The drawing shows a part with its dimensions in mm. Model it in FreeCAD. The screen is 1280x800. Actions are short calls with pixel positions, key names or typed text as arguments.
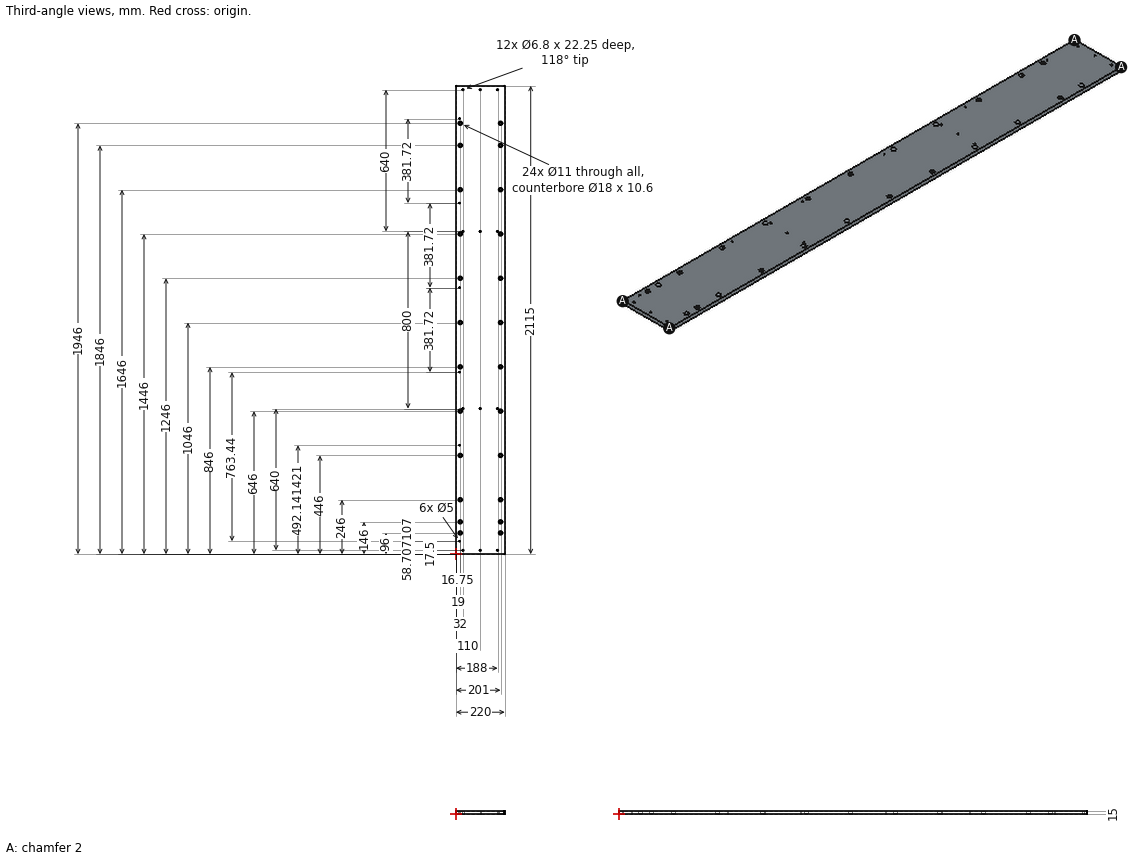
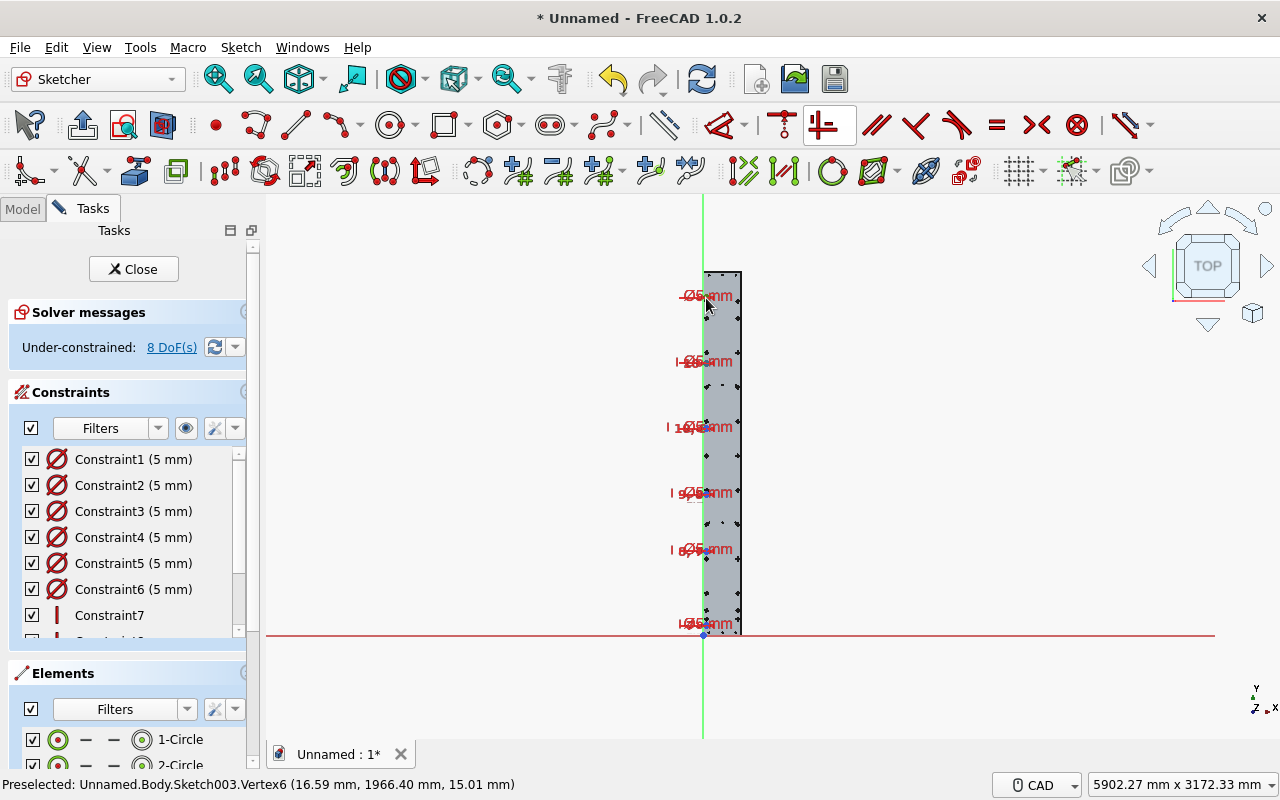
key(v)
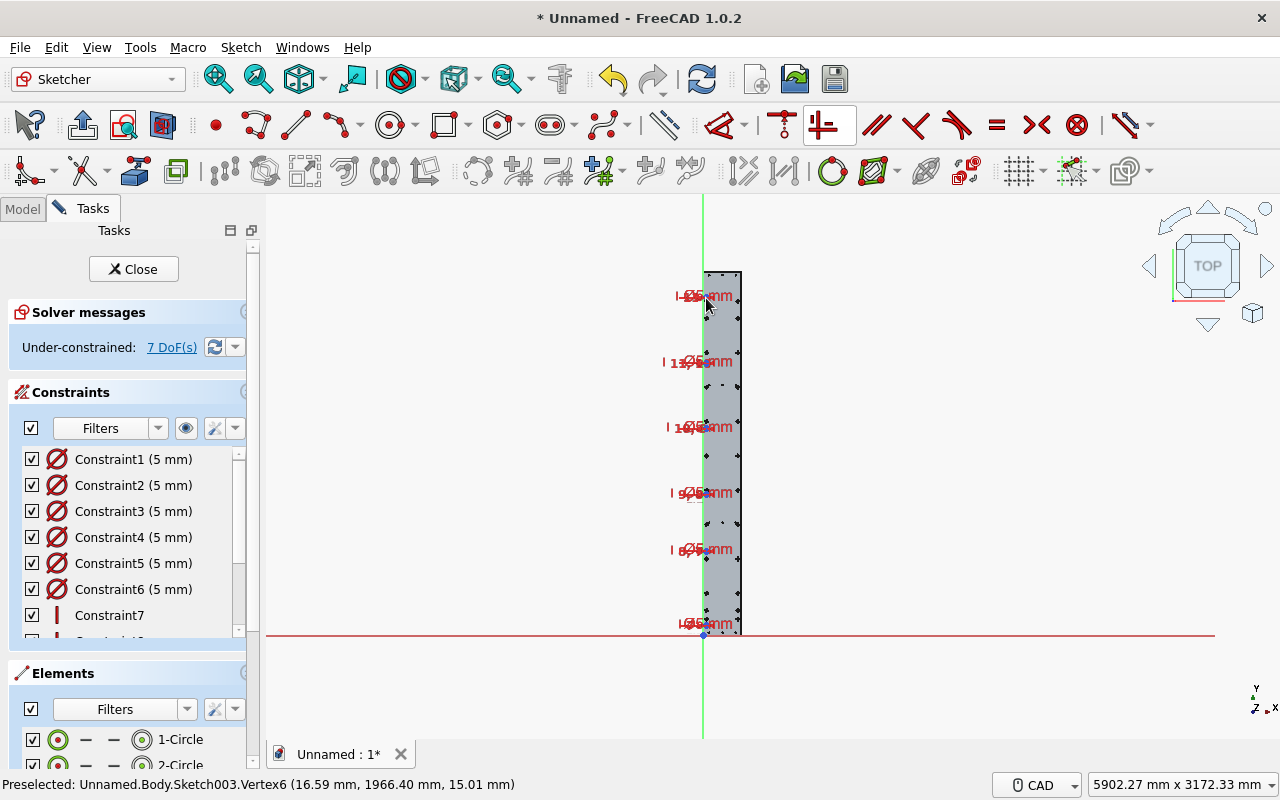
click(720, 126)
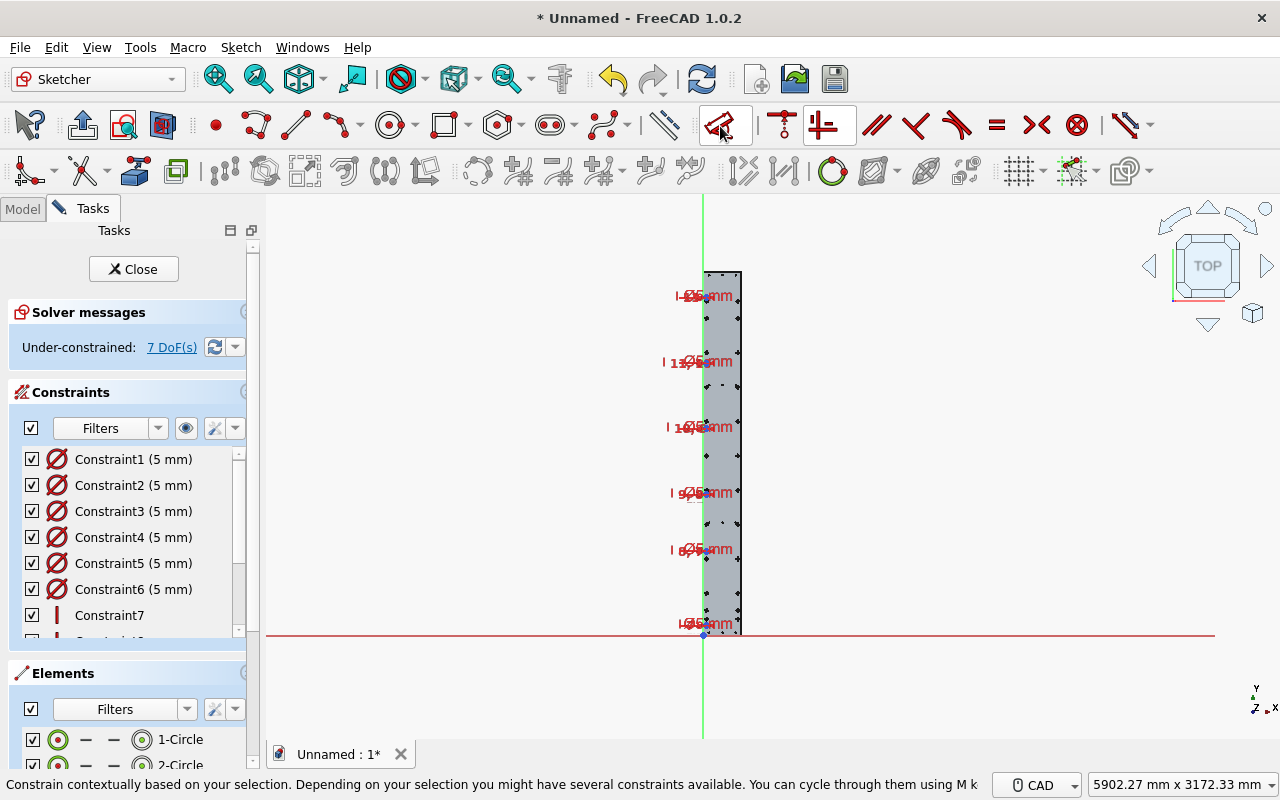
scroll(706, 626, up, 14)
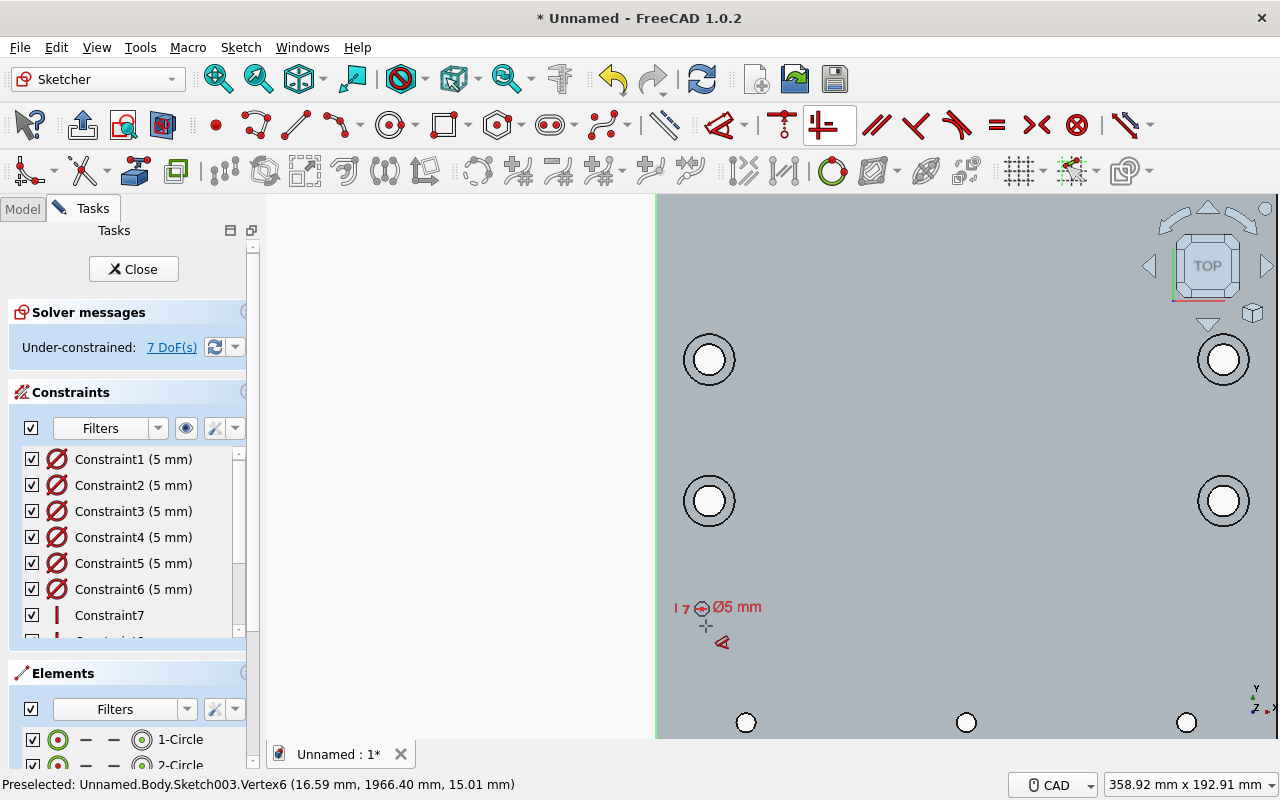
click(702, 609)
click(679, 575)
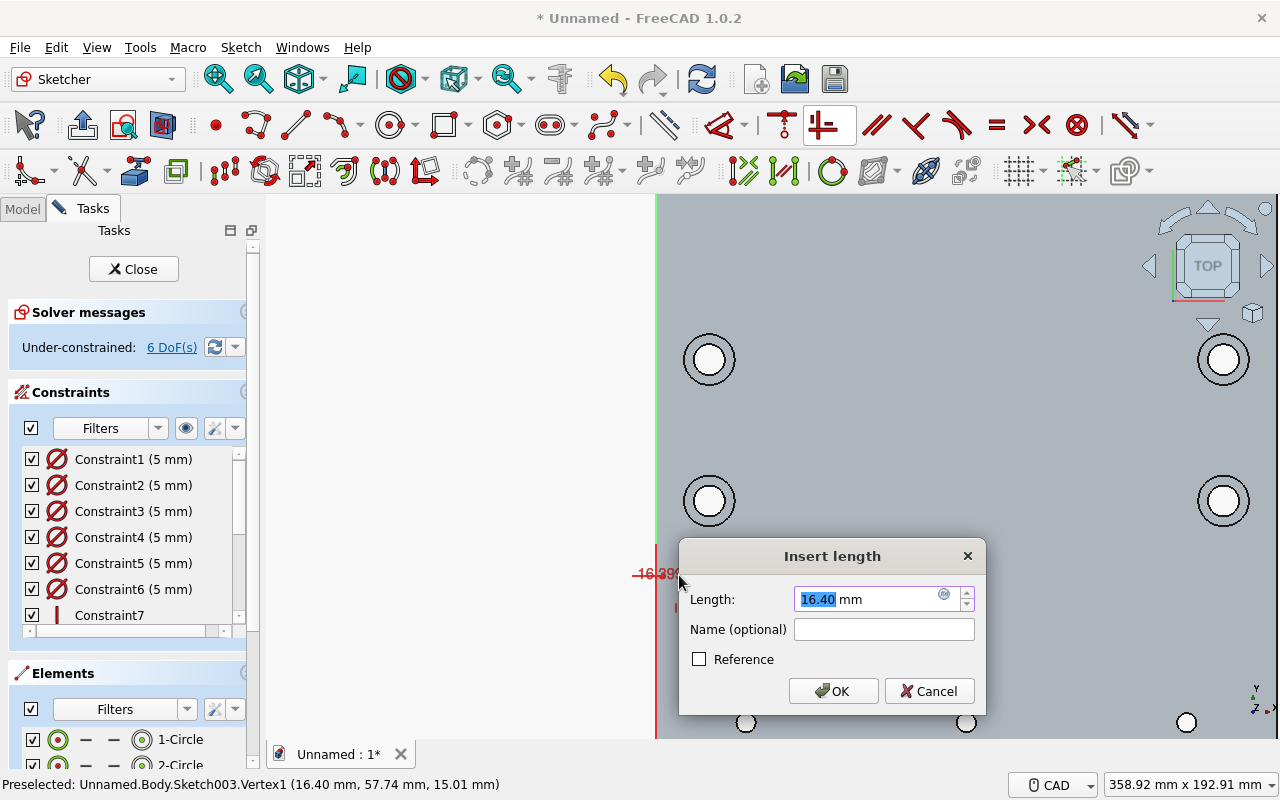
text(16.75)
key(Return)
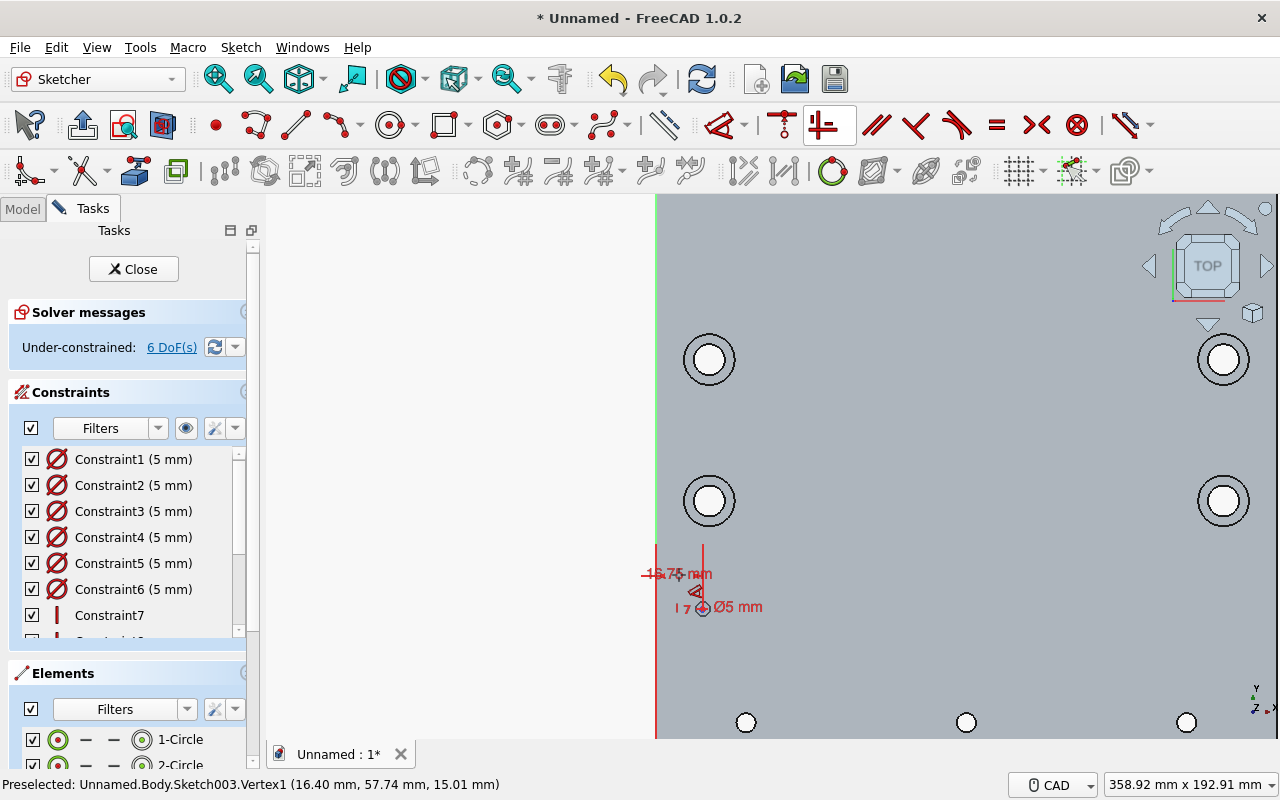
scroll(706, 627, down, 14)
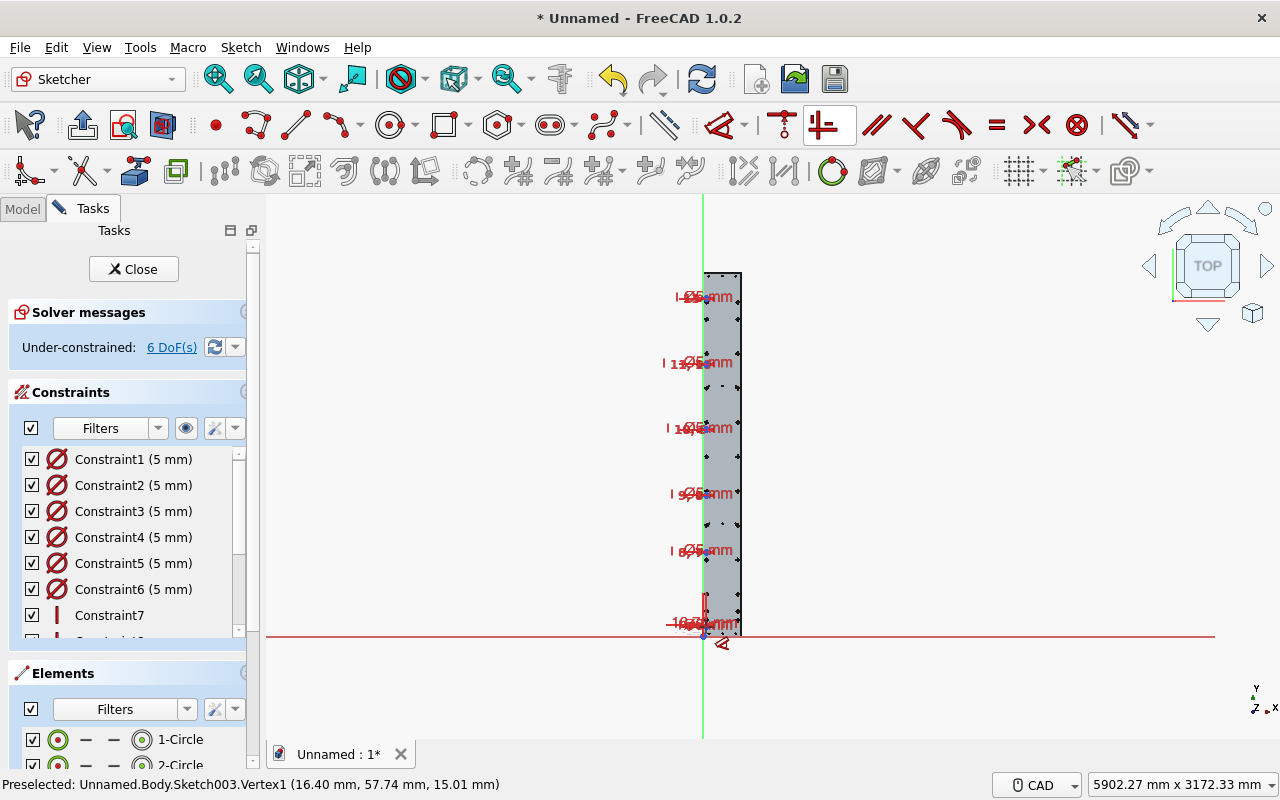
click(706, 627)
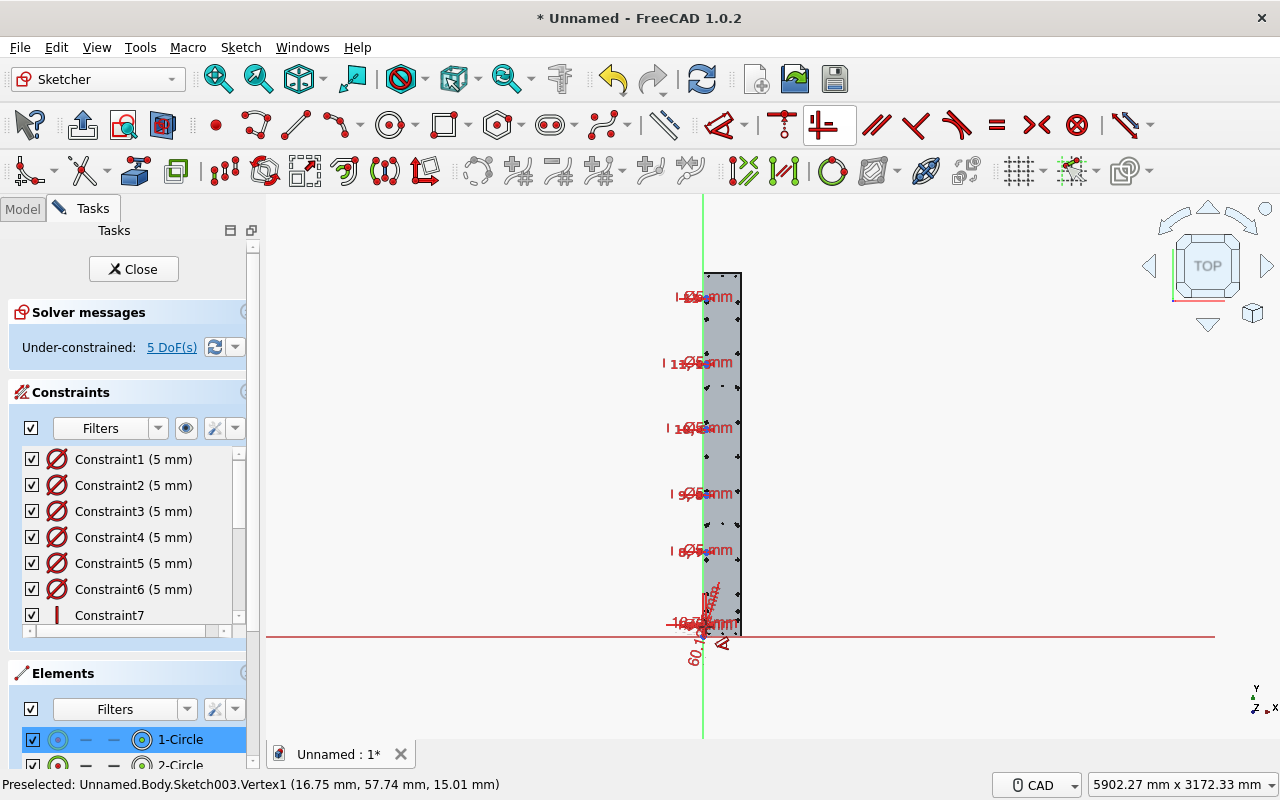
click(706, 495)
click(740, 561)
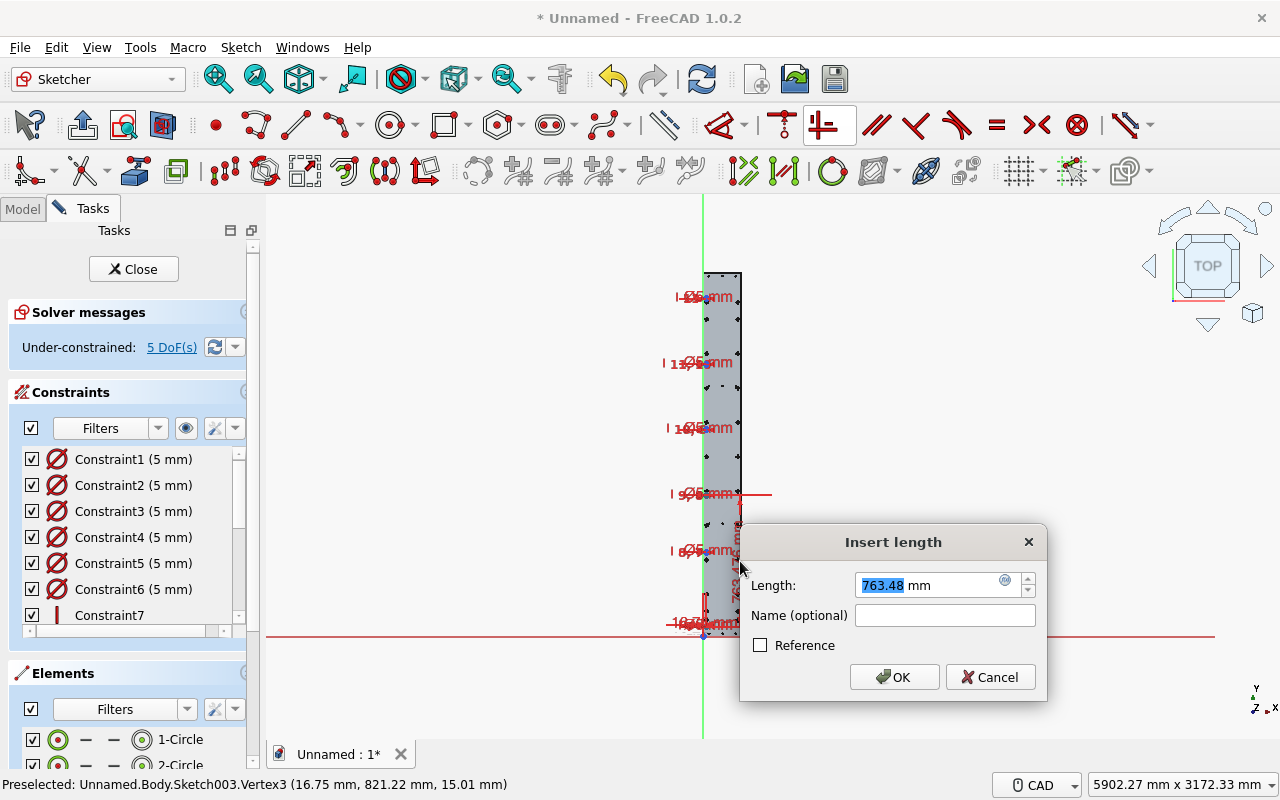
text(763.44)
key(Return)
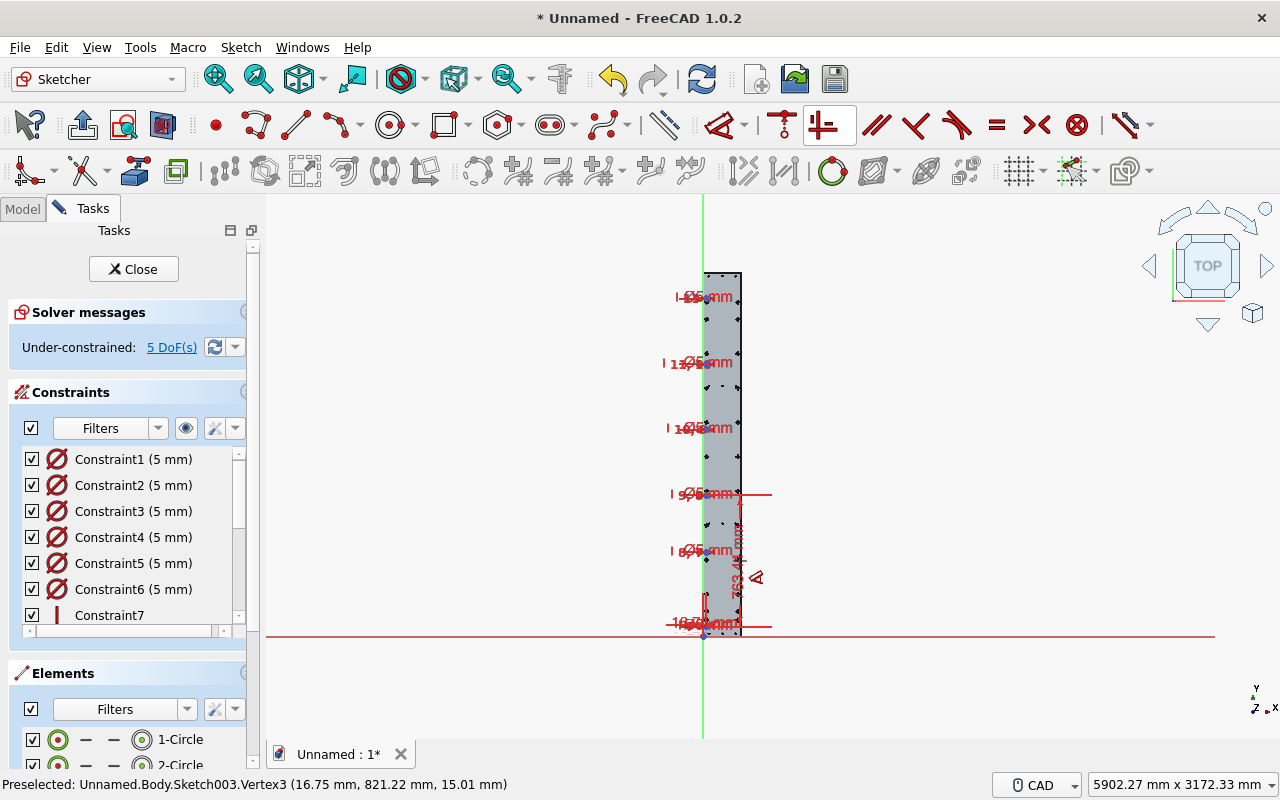
click(706, 495)